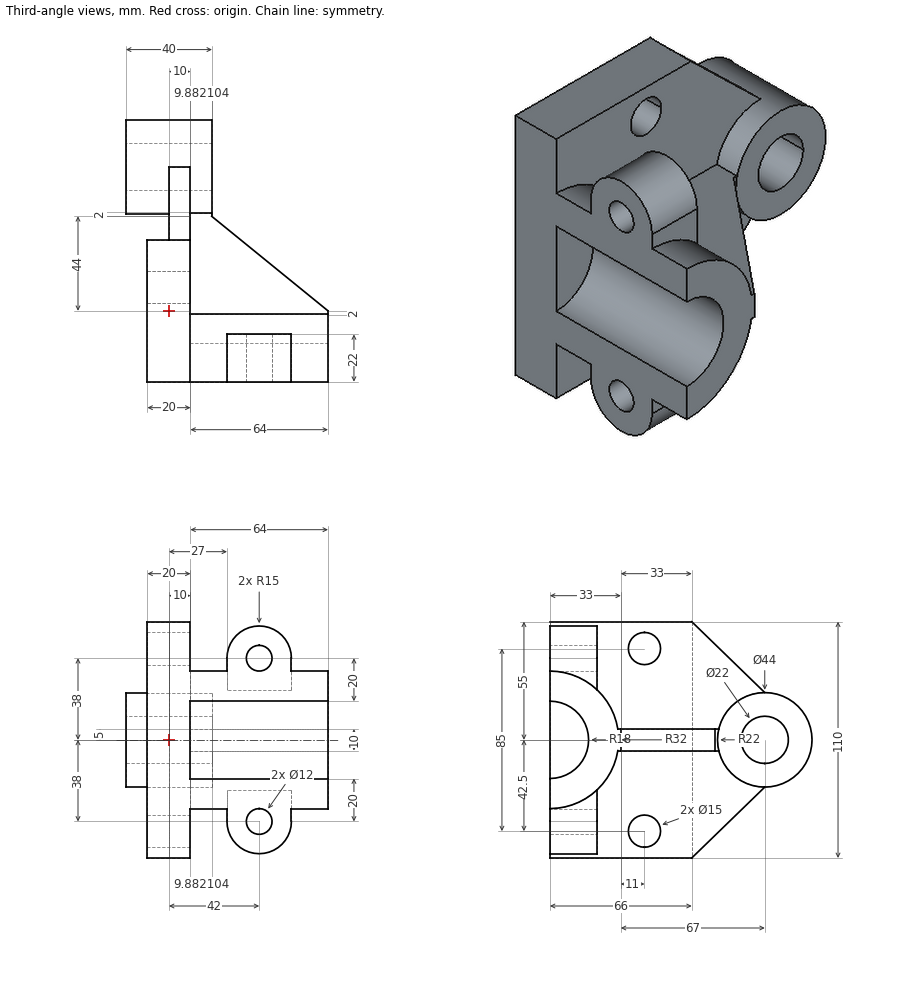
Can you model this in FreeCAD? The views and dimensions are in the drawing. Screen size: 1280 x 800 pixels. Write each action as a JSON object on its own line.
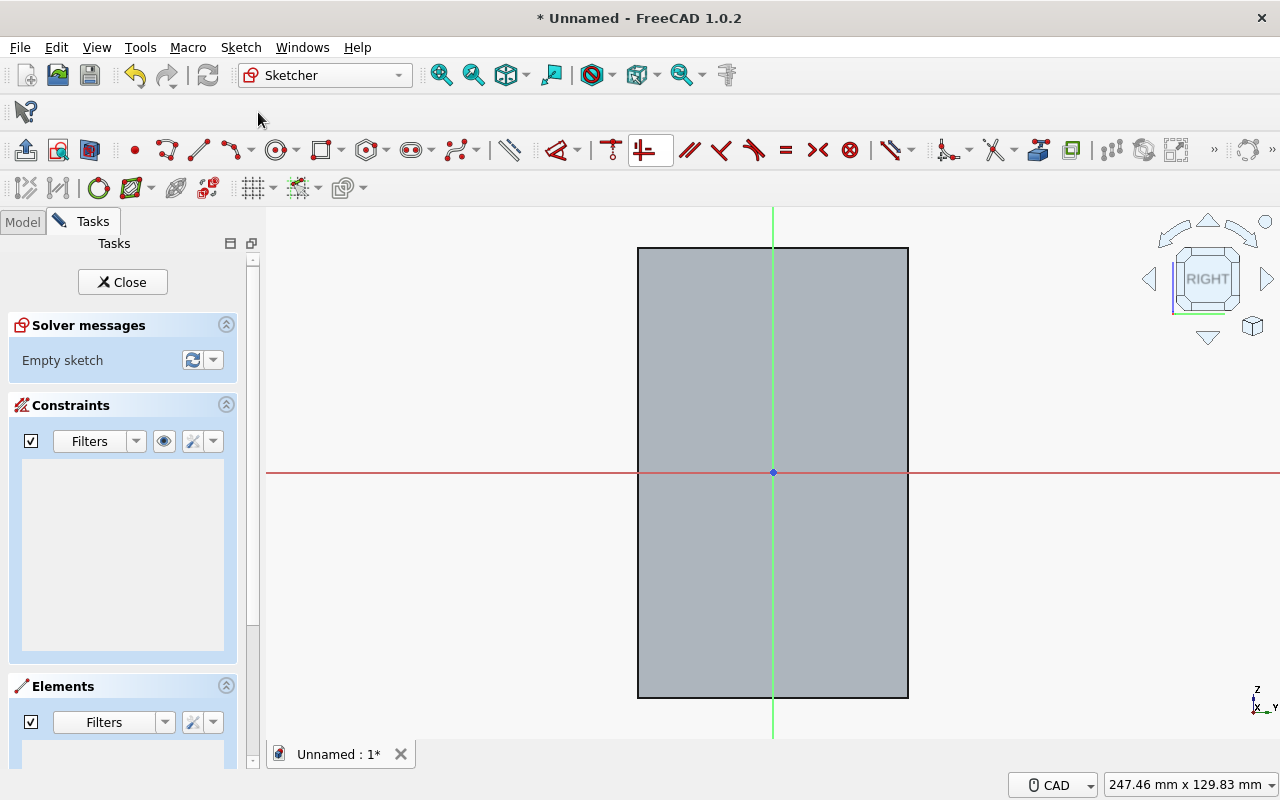
{"action": "key", "text": "g c"}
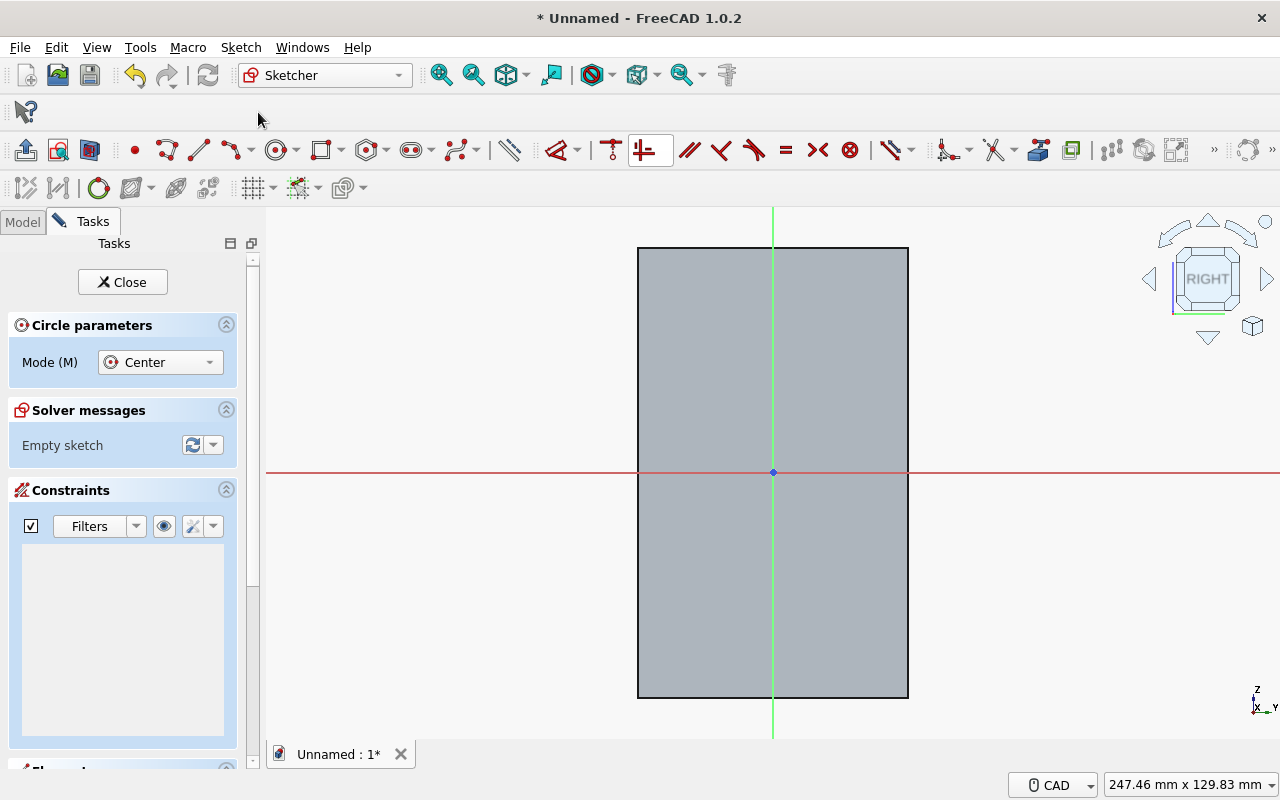
{"action": "left_click", "coordinate": [818, 647]}
{"action": "left_click", "coordinate": [840, 625]}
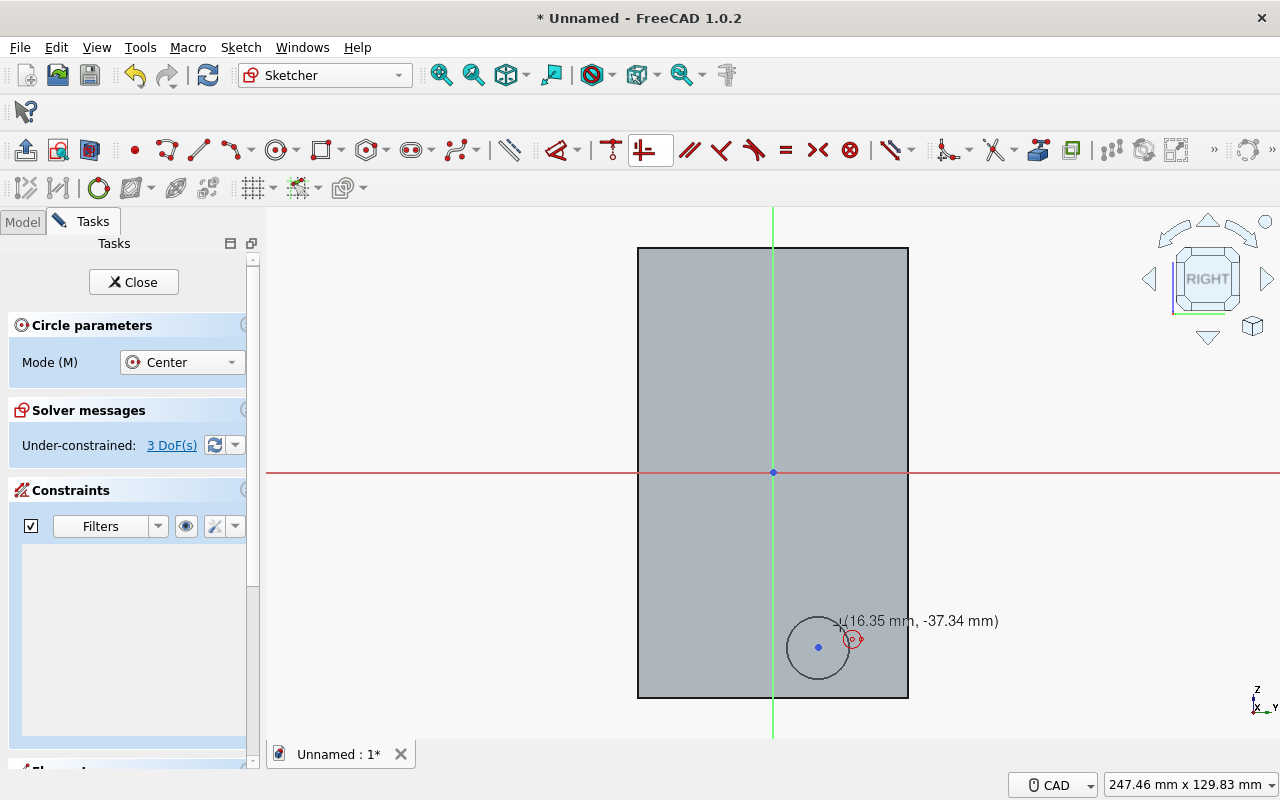
{"action": "left_click", "coordinate": [818, 299]}
{"action": "left_click", "coordinate": [840, 277]}
{"action": "key", "text": "Escape"}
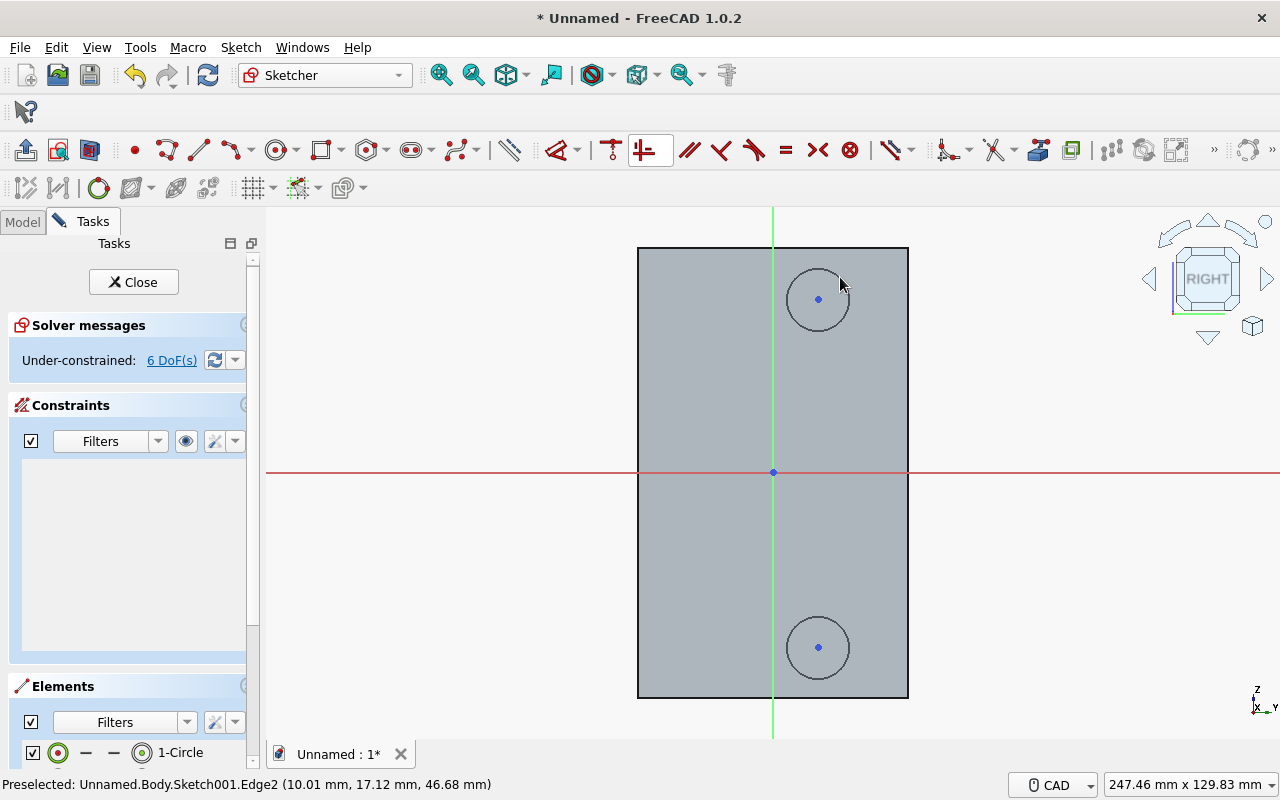
{"action": "left_click", "coordinate": [840, 626]}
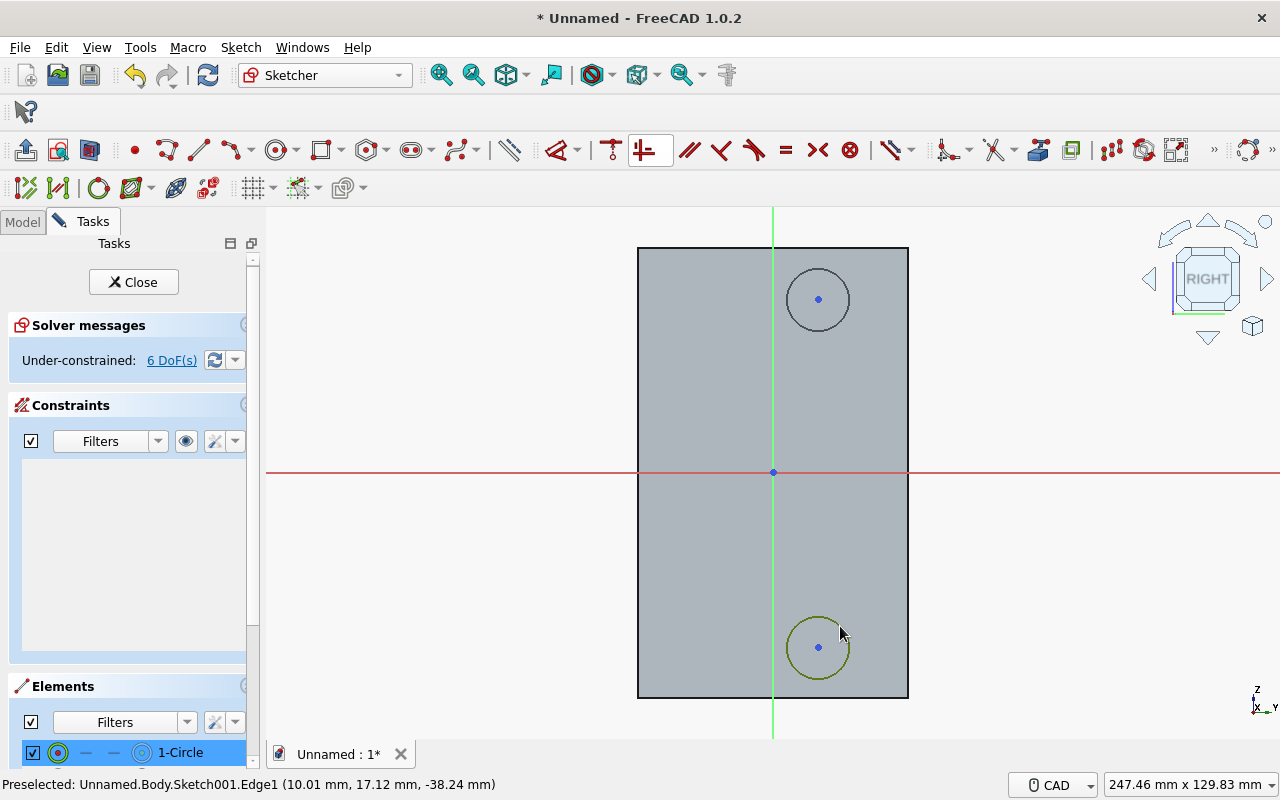
{"action": "left_click", "coordinate": [840, 278]}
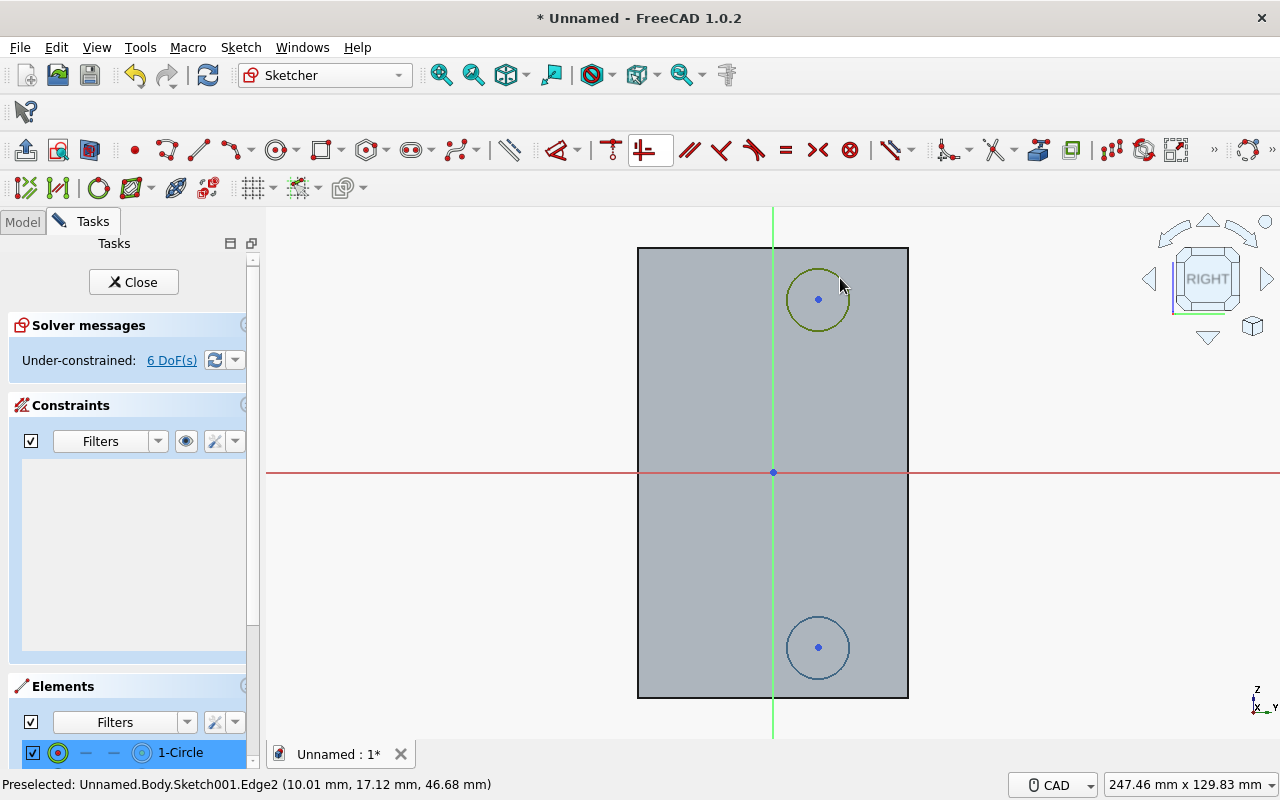
{"action": "left_click", "coordinate": [786, 150]}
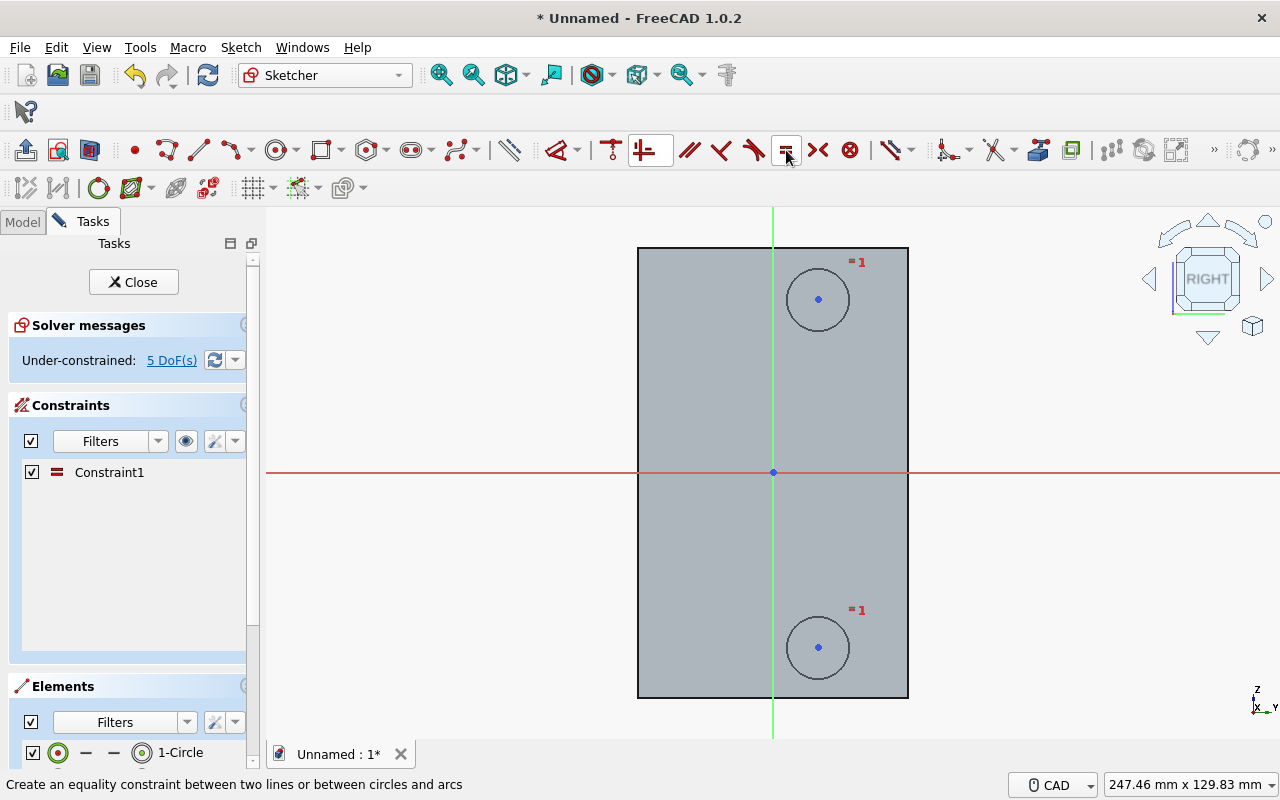
{"action": "left_click", "coordinate": [818, 648]}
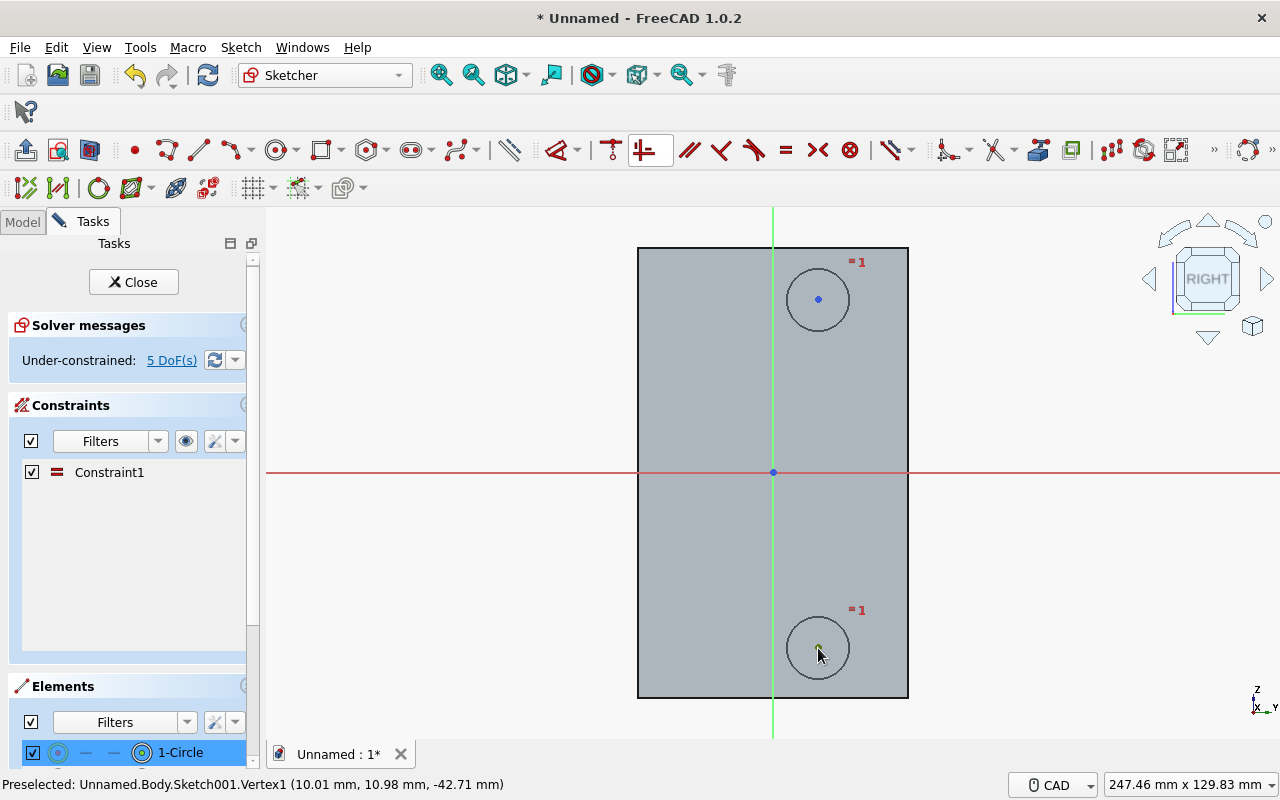
{"action": "left_click", "coordinate": [818, 300]}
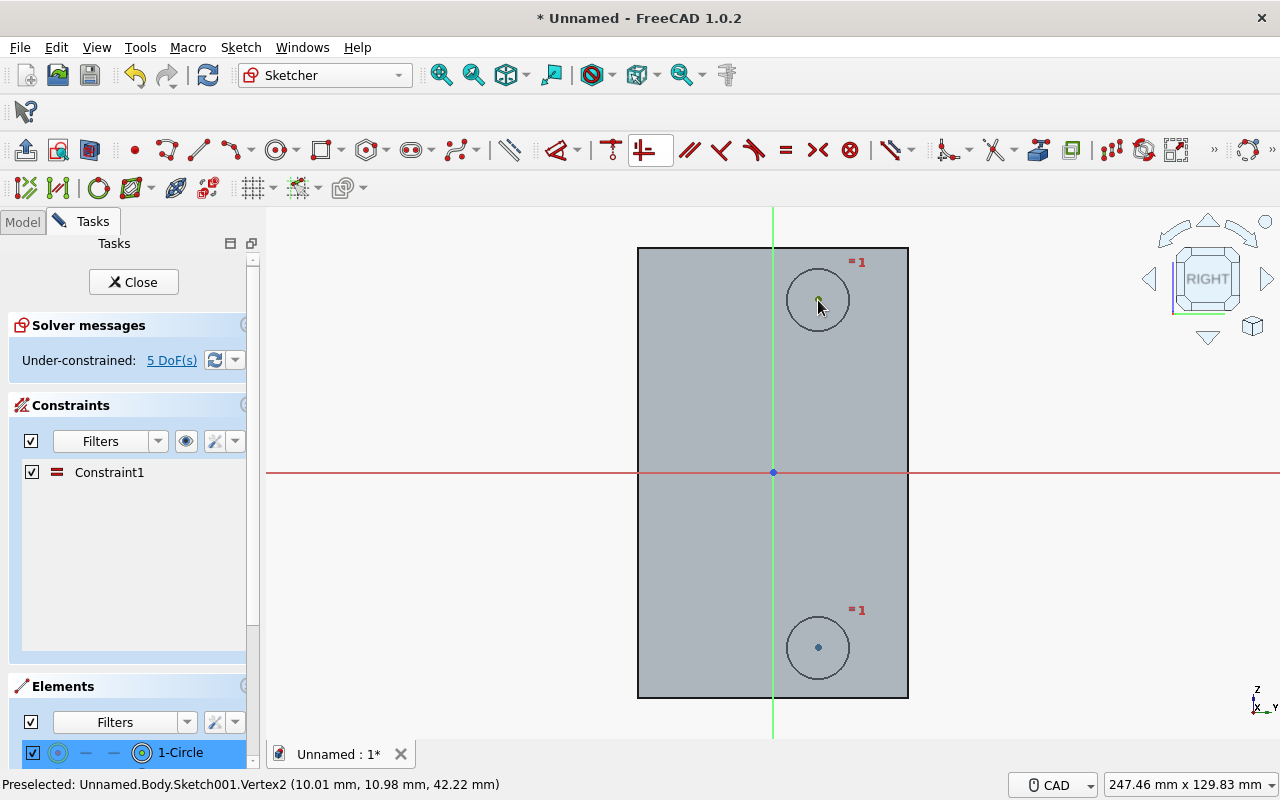
{"action": "key", "text": "v"}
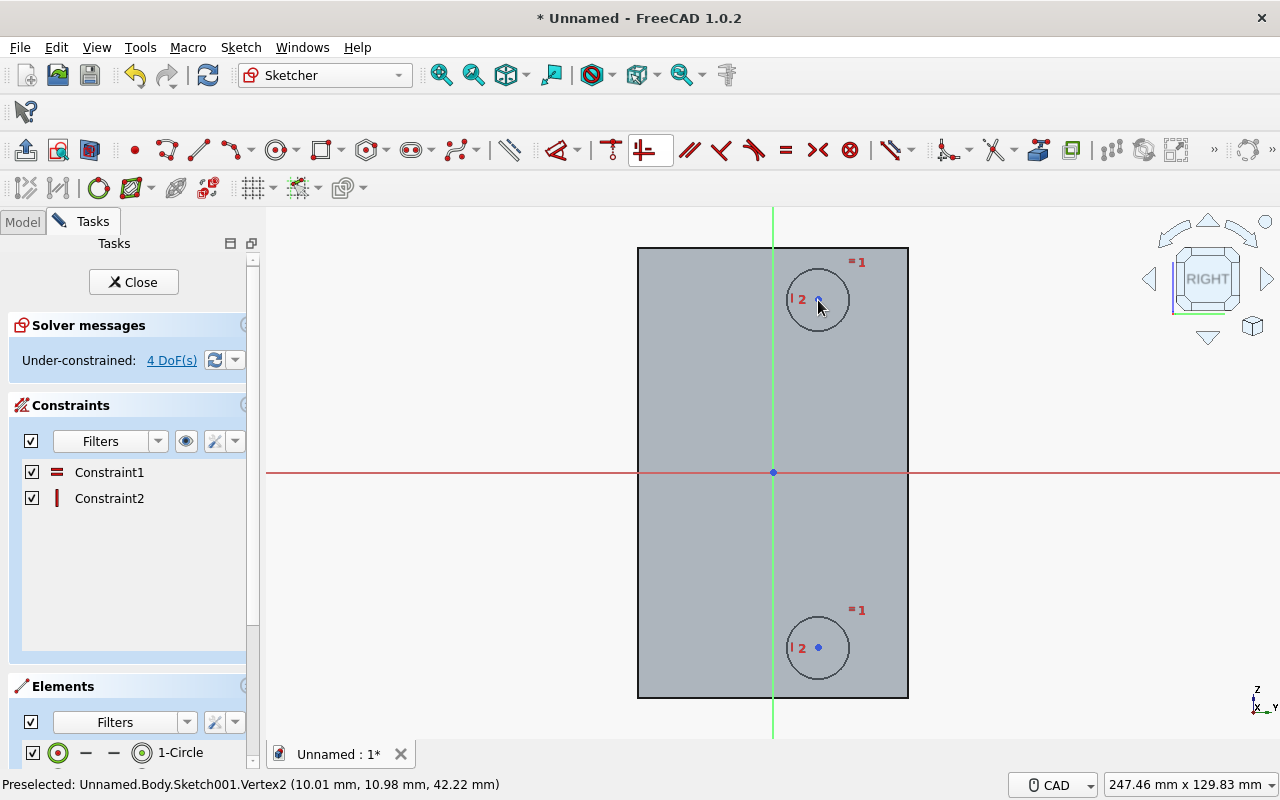
{"action": "left_click", "coordinate": [556, 150]}